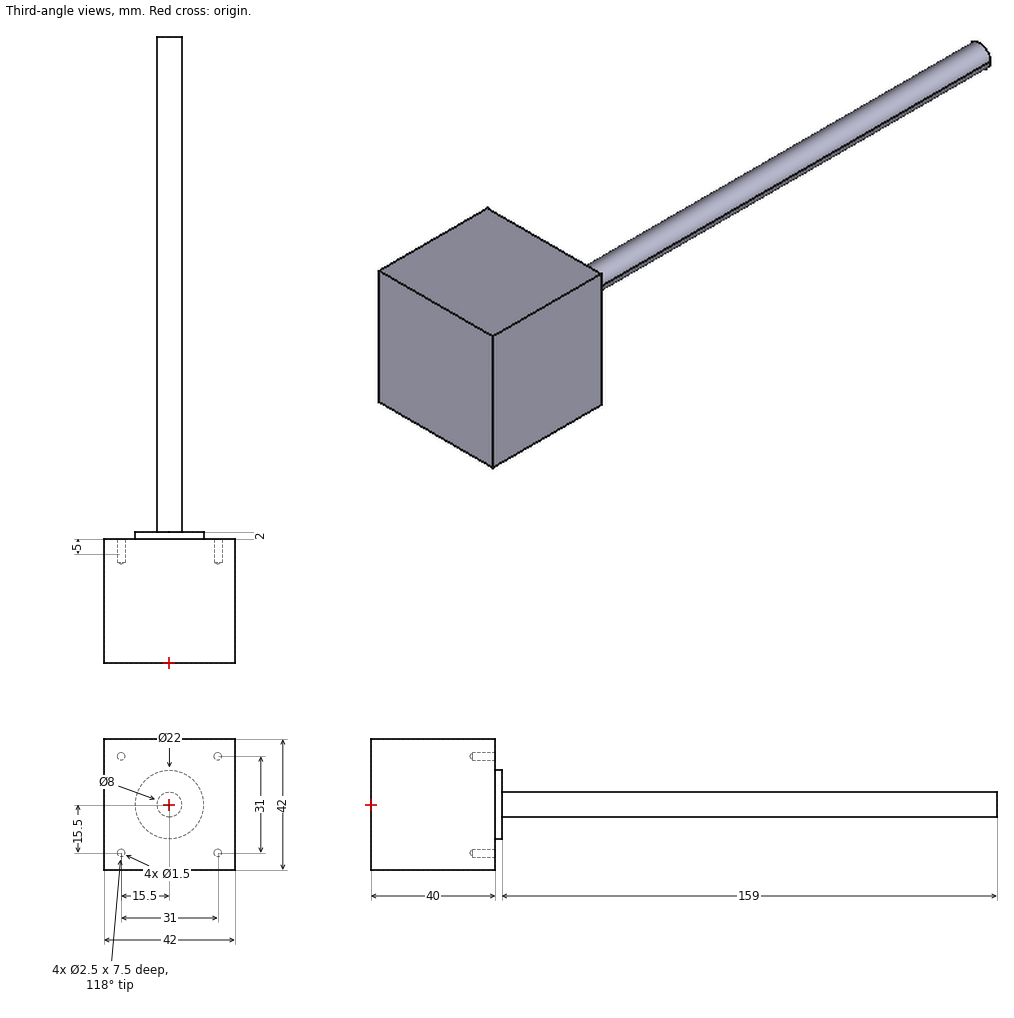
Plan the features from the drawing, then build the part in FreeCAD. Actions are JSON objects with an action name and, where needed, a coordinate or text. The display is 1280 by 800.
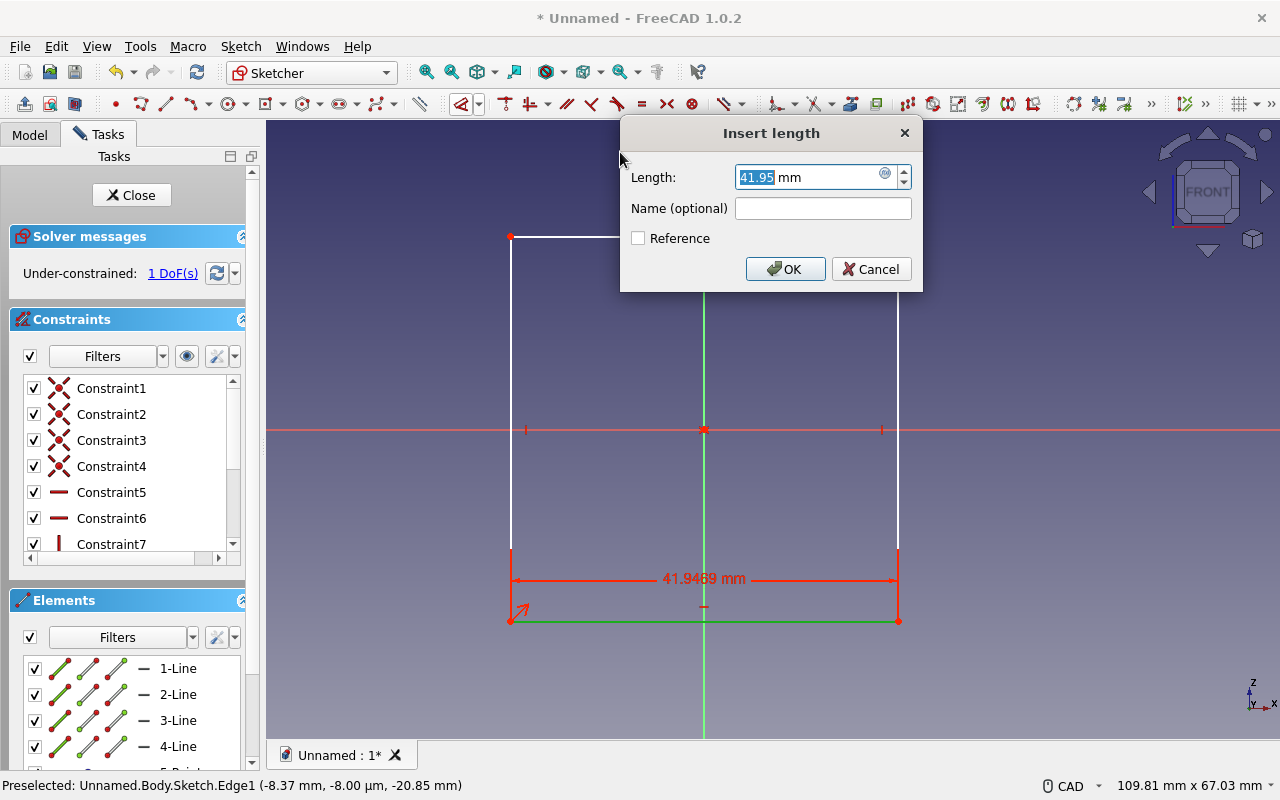
{"action": "type", "text": "42"}
{"action": "key", "text": "Return"}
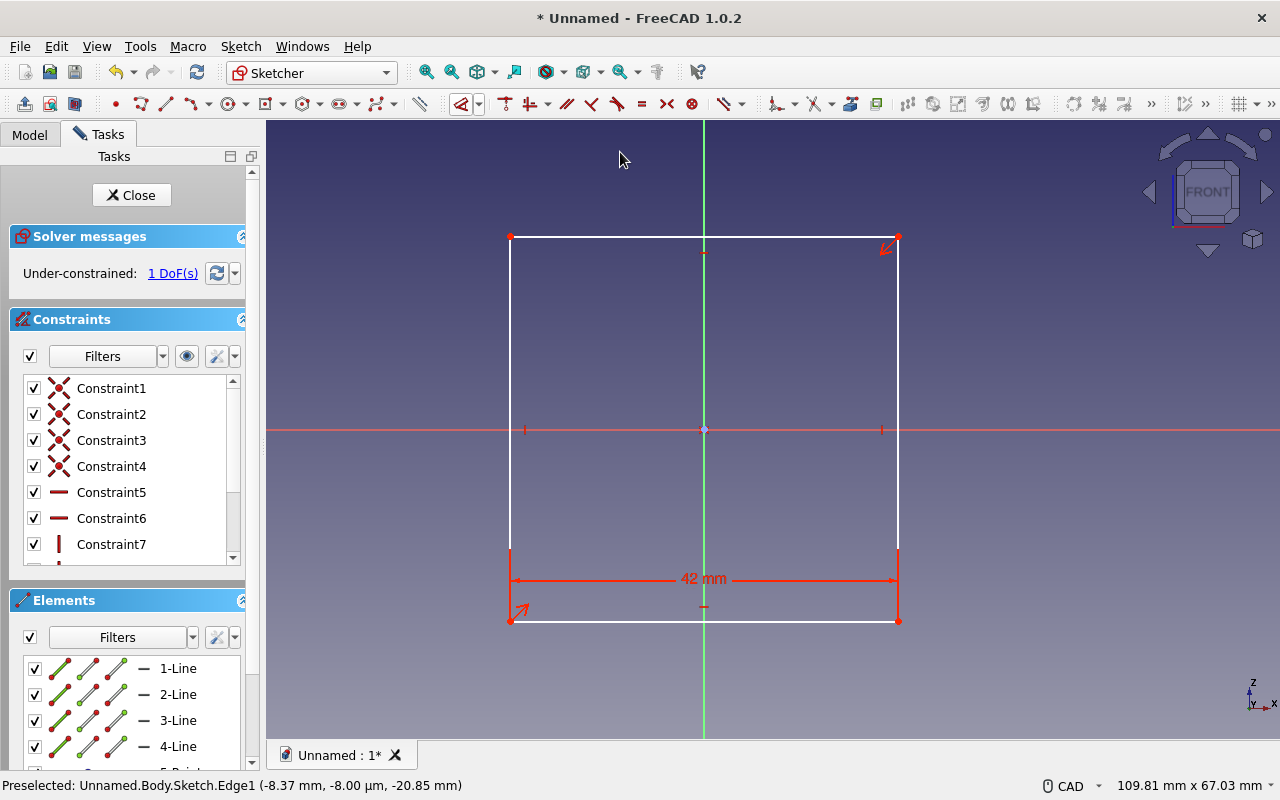
{"action": "left_click", "coordinate": [898, 506]}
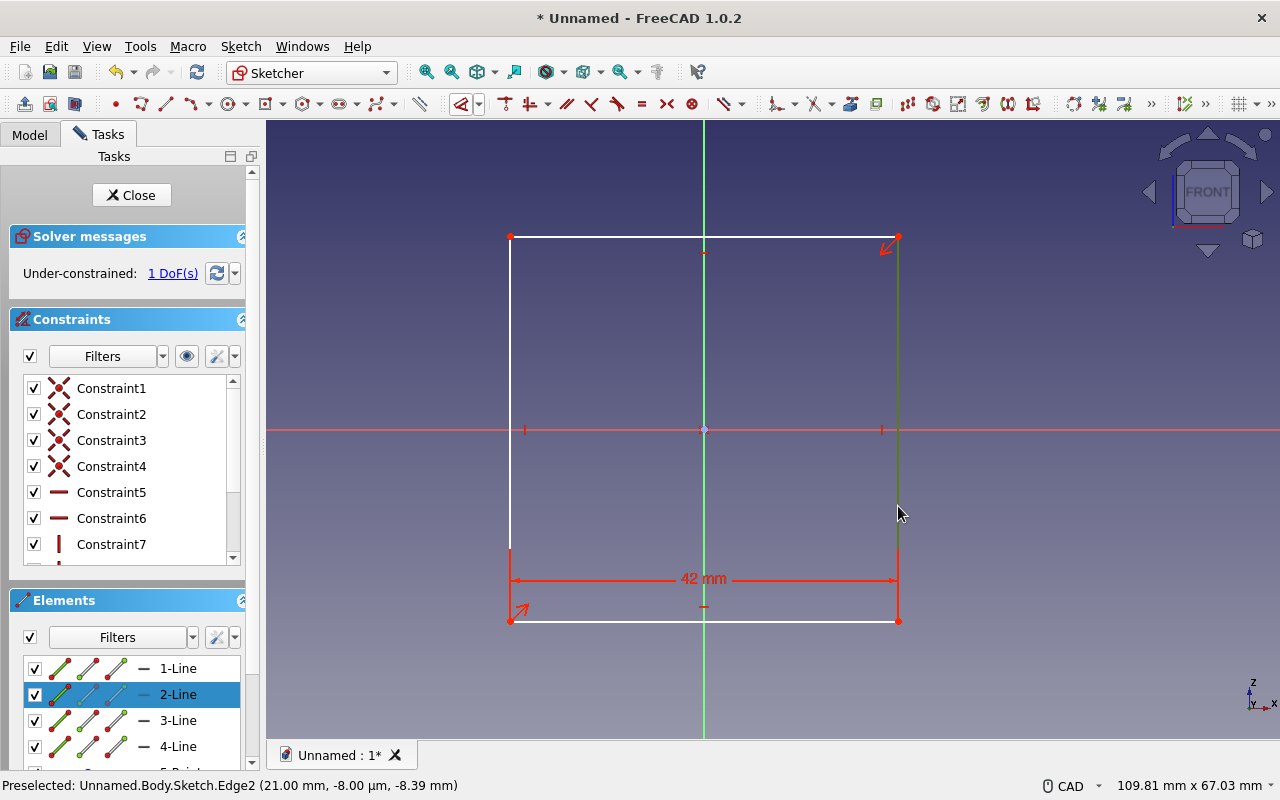
{"action": "key", "text": "i"}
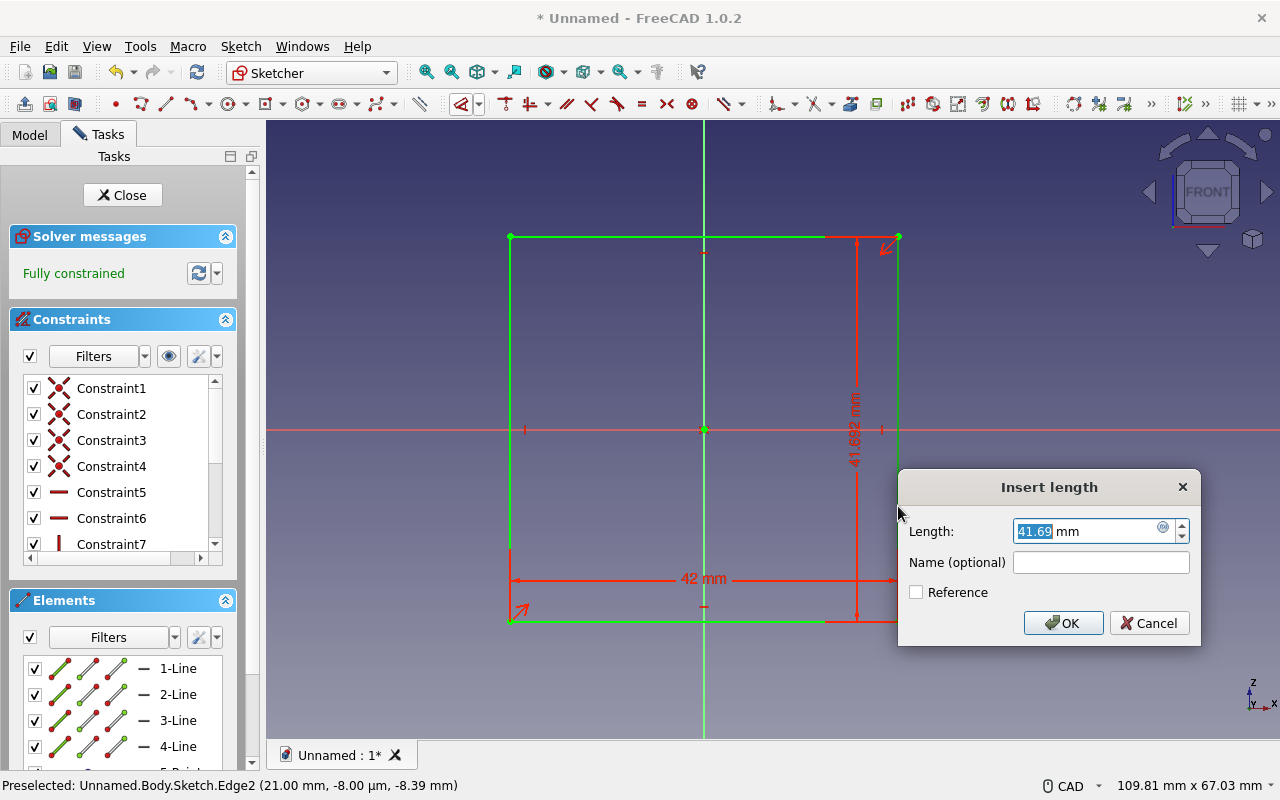
{"action": "type", "text": "42"}
{"action": "key", "text": "Return"}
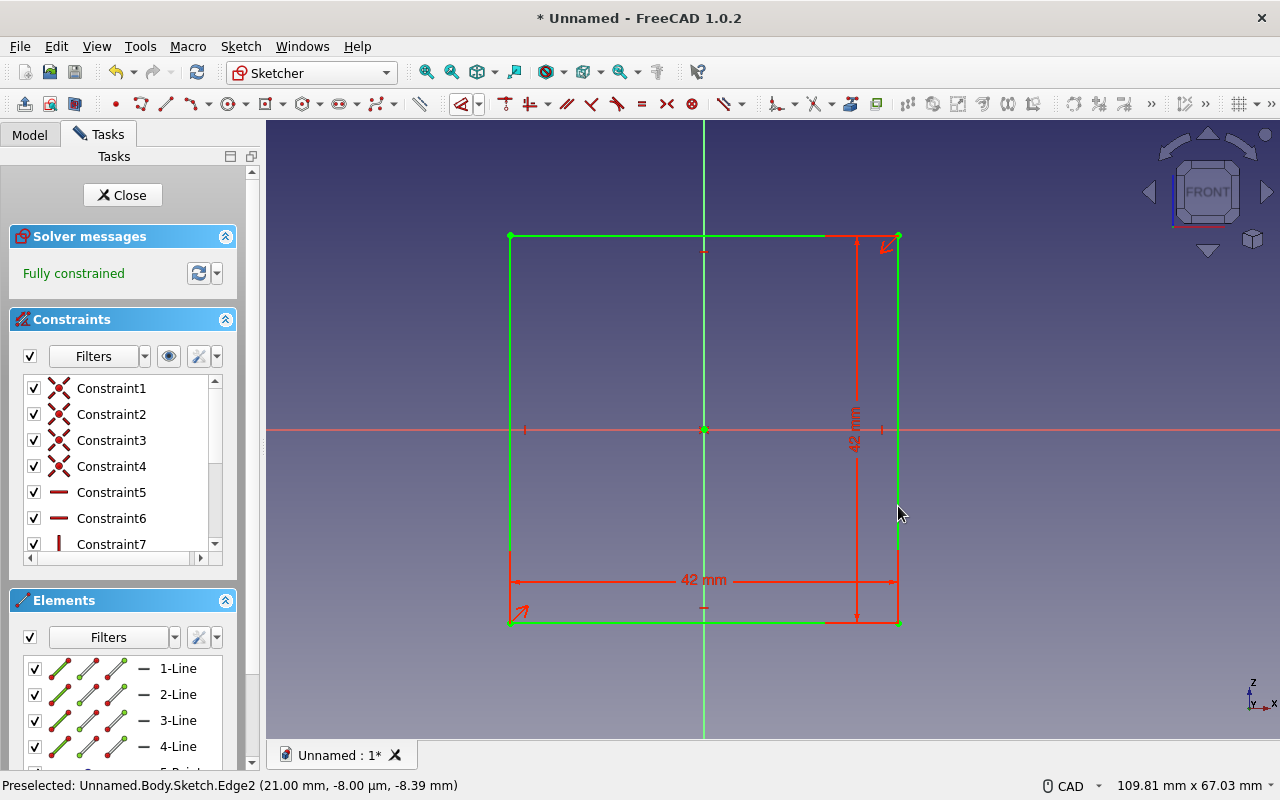
{"action": "left_click", "coordinate": [123, 195]}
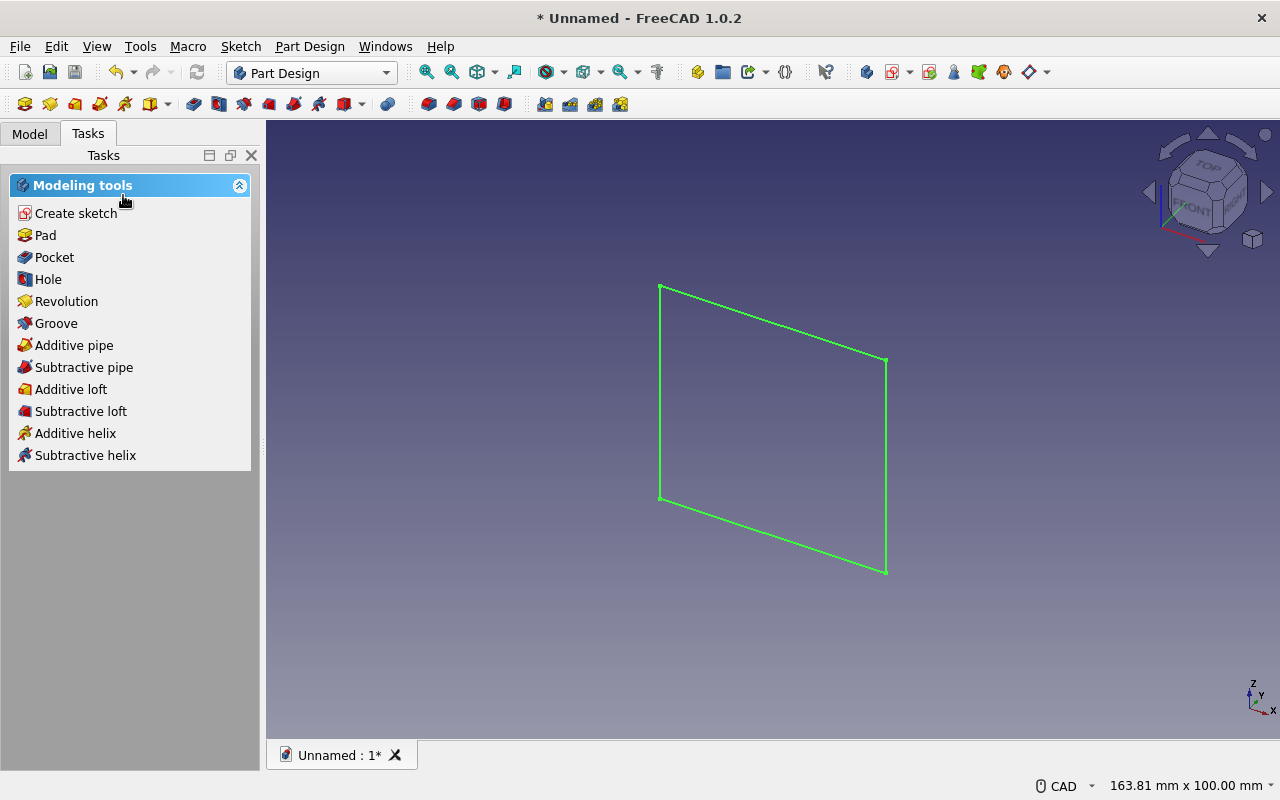
{"action": "left_click", "coordinate": [25, 104]}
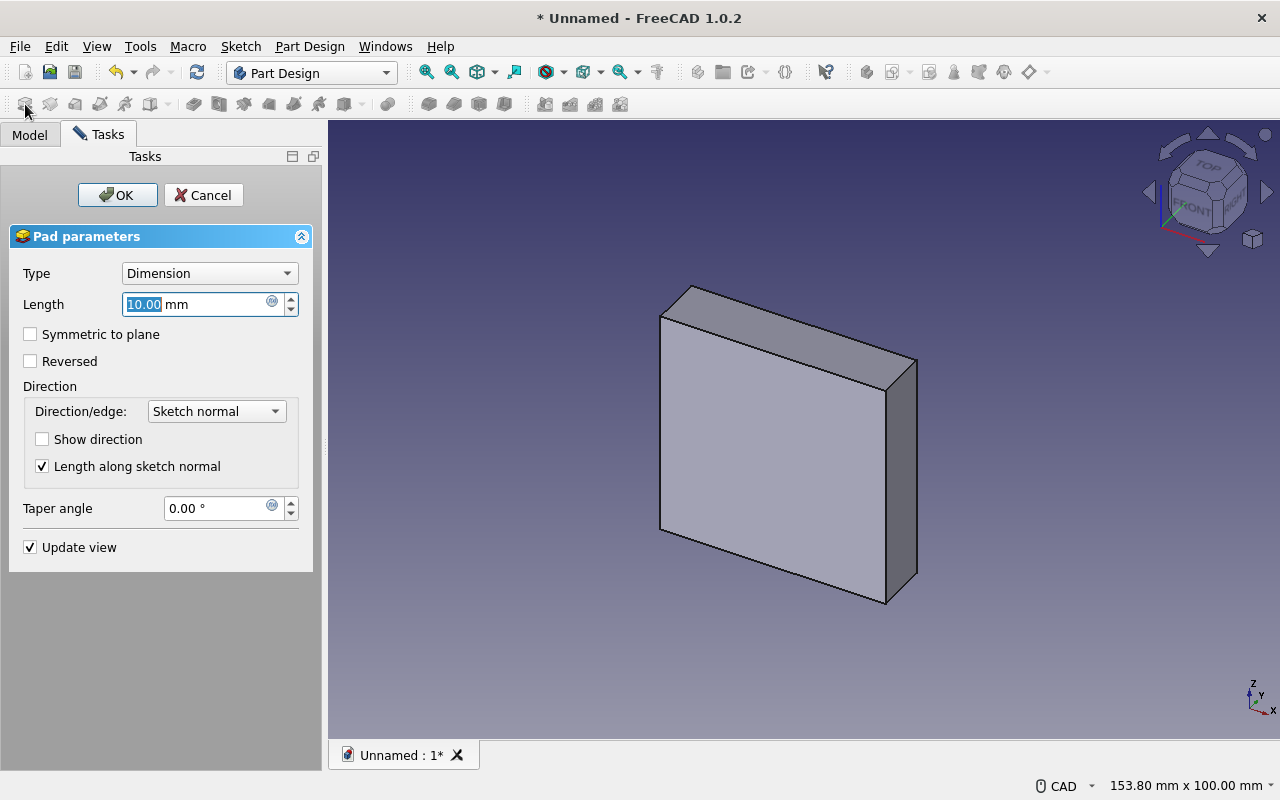
{"action": "type", "text": "40"}
{"action": "key", "text": "Tab"}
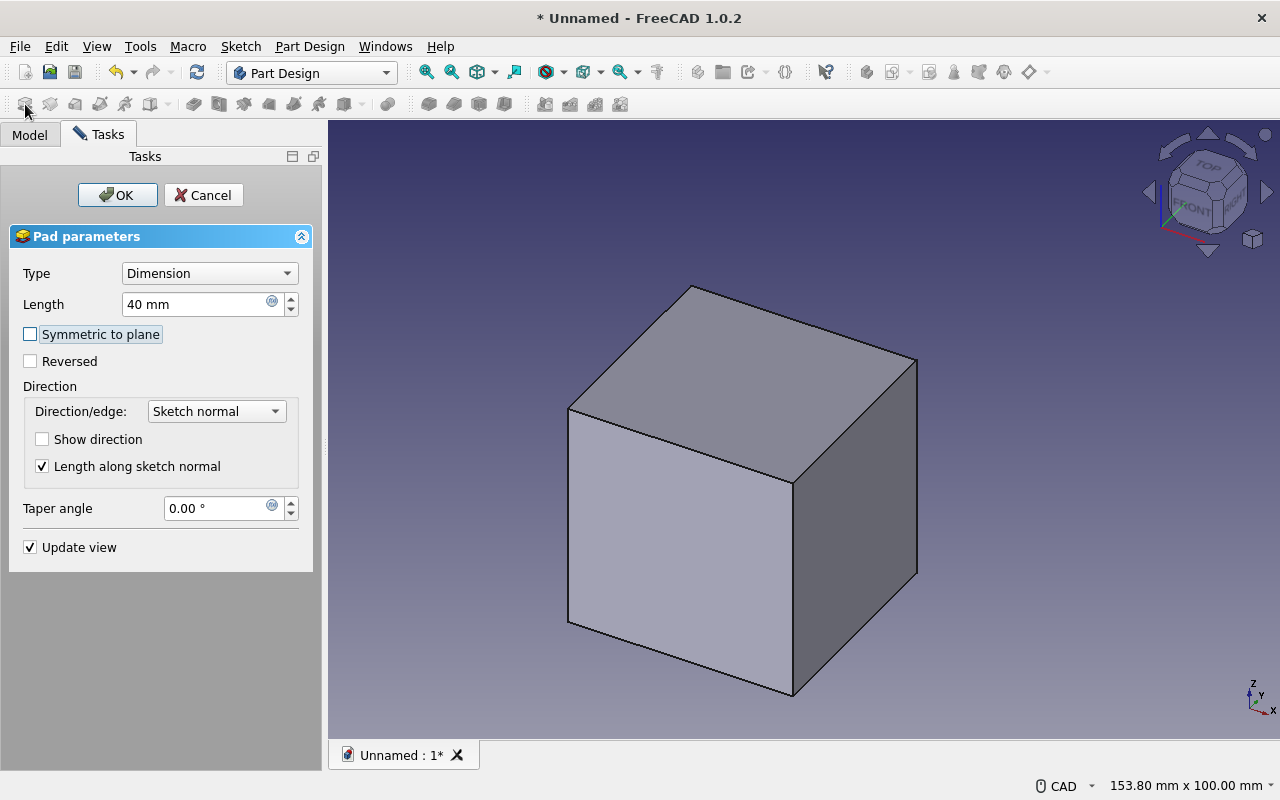
{"action": "left_click", "coordinate": [31, 361]}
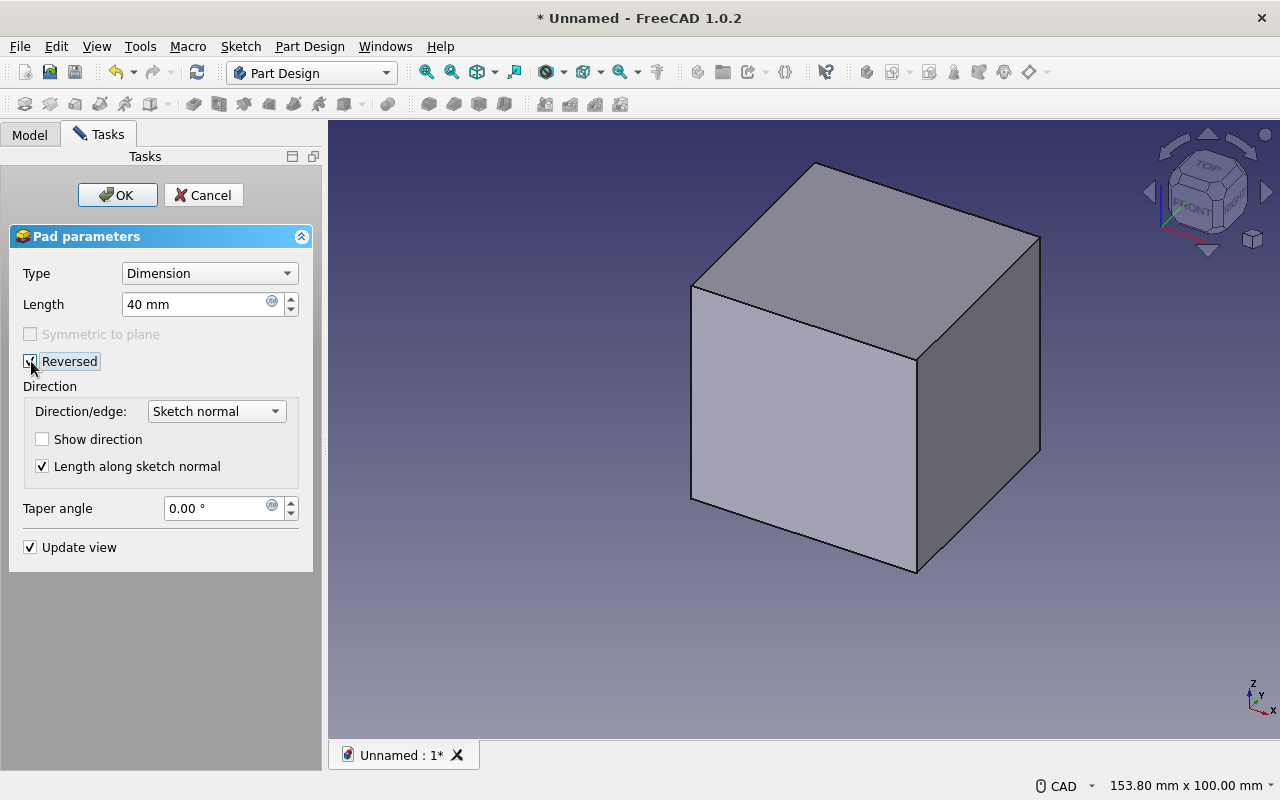
{"action": "left_click", "coordinate": [118, 195]}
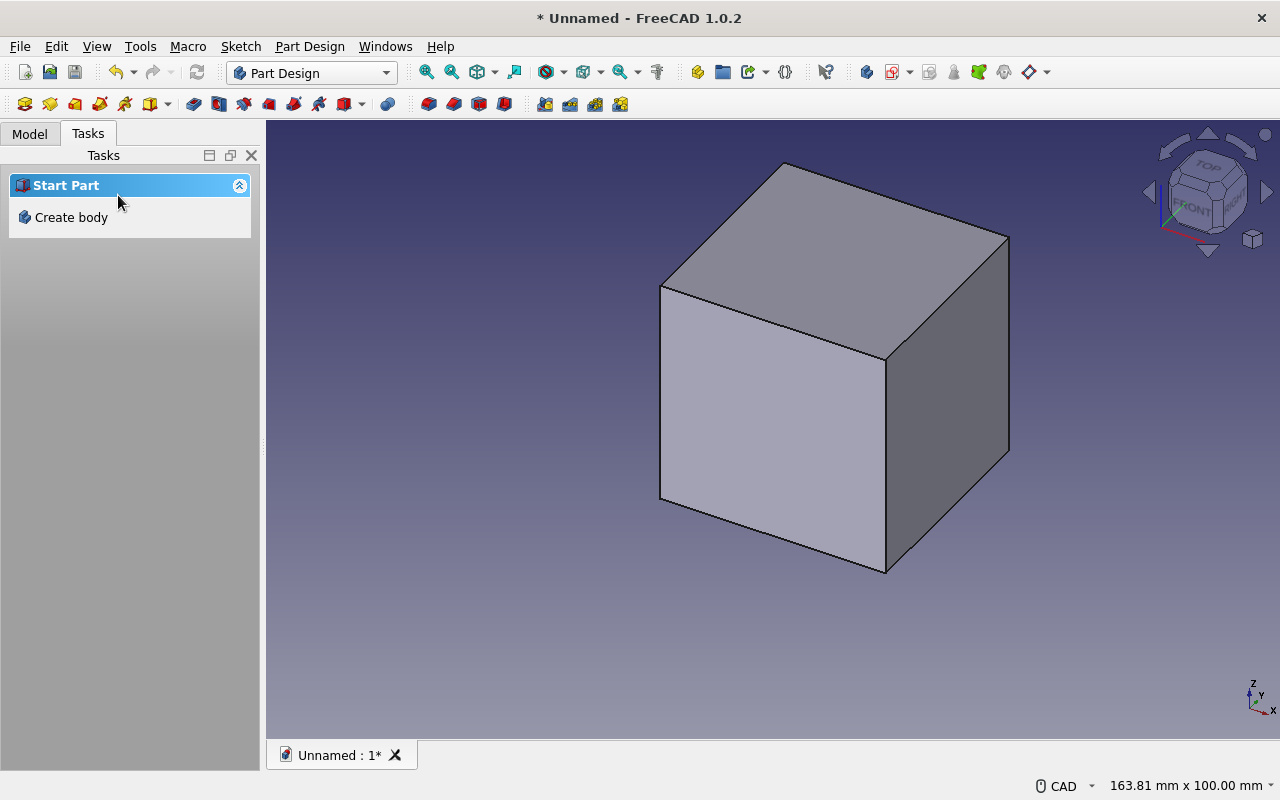
{"action": "key", "text": "4"}